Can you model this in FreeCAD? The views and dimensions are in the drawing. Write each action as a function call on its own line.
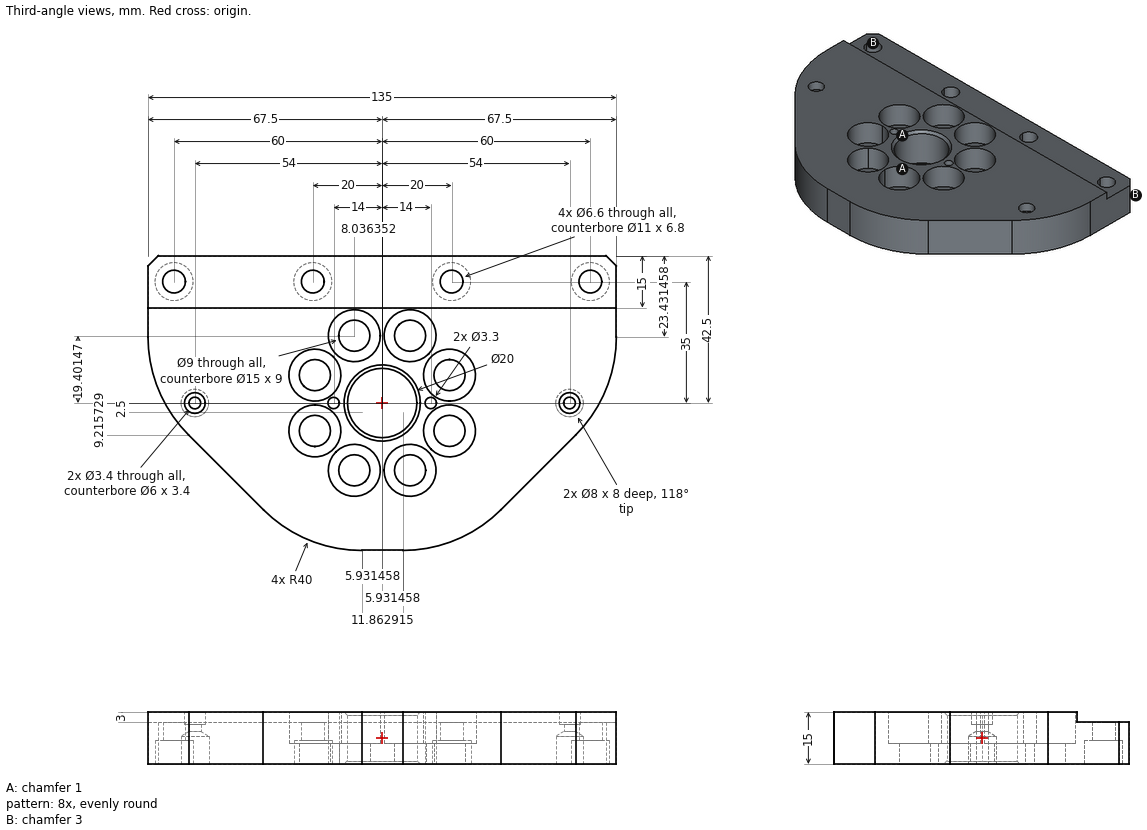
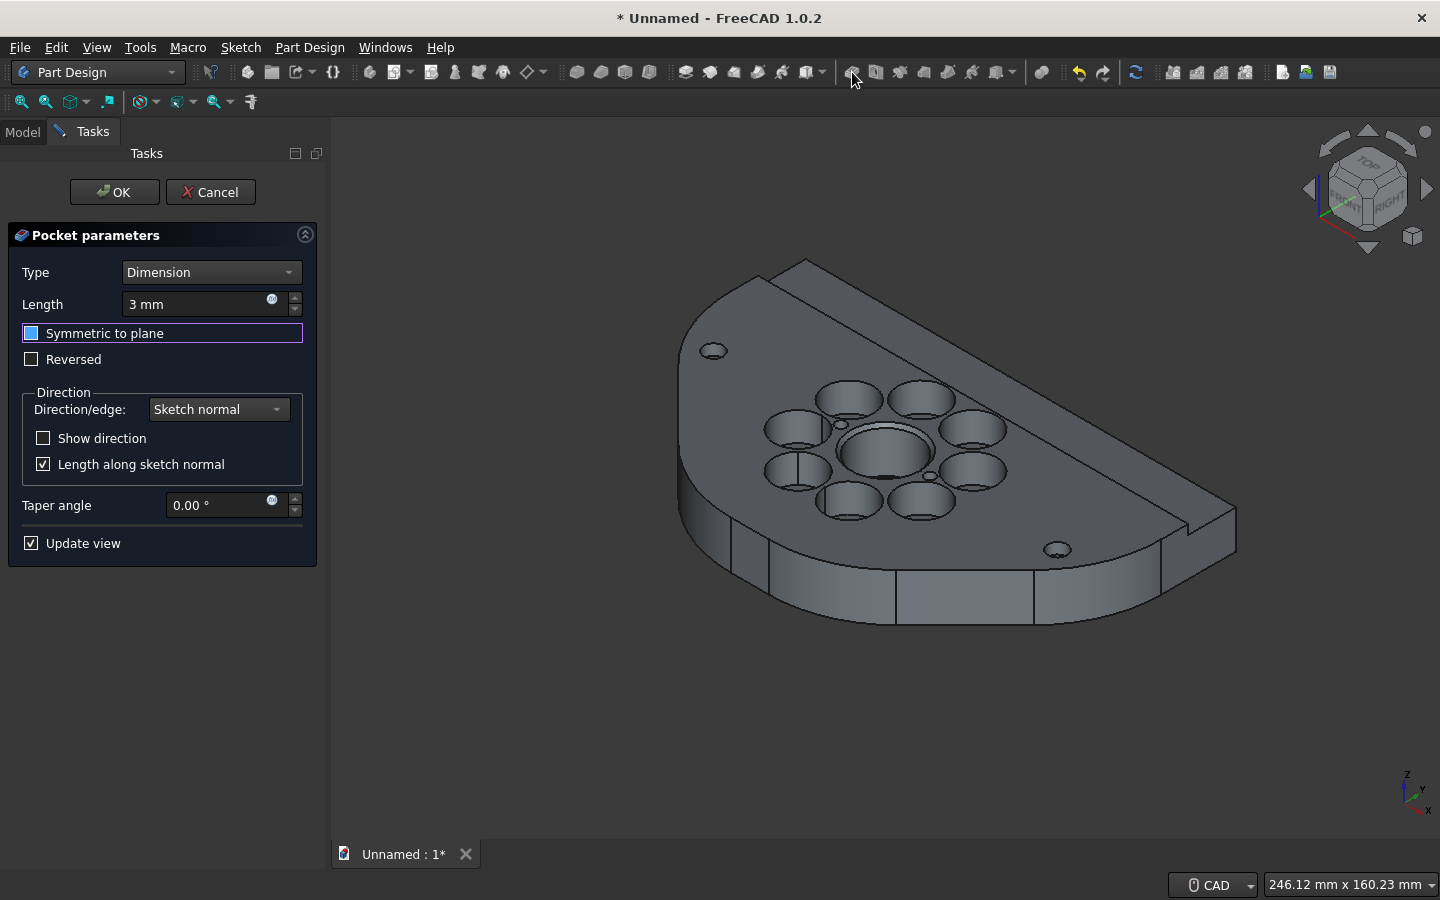
click(115, 192)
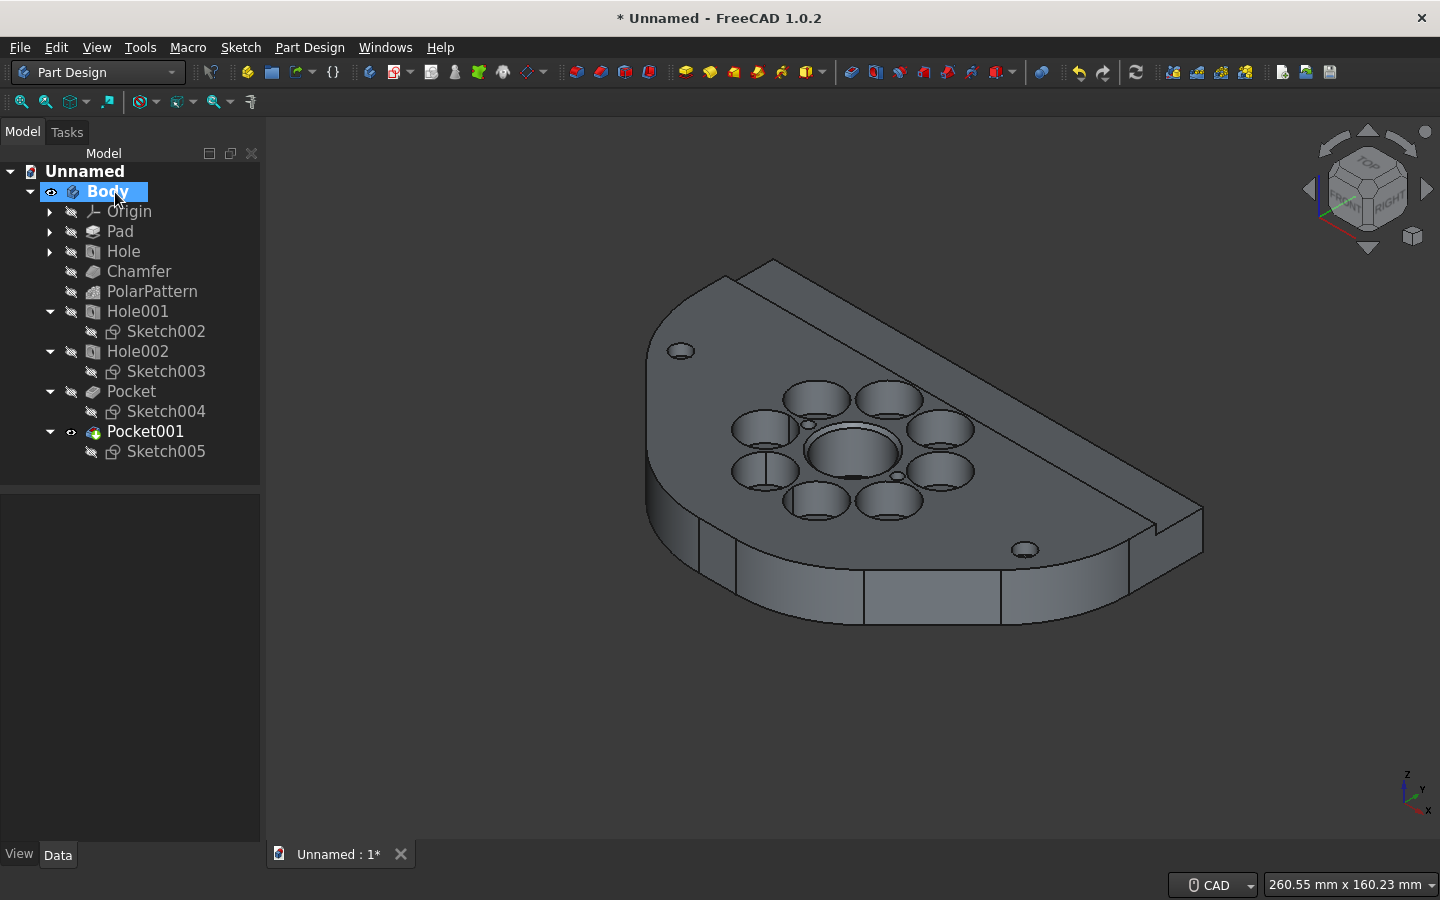
key(5)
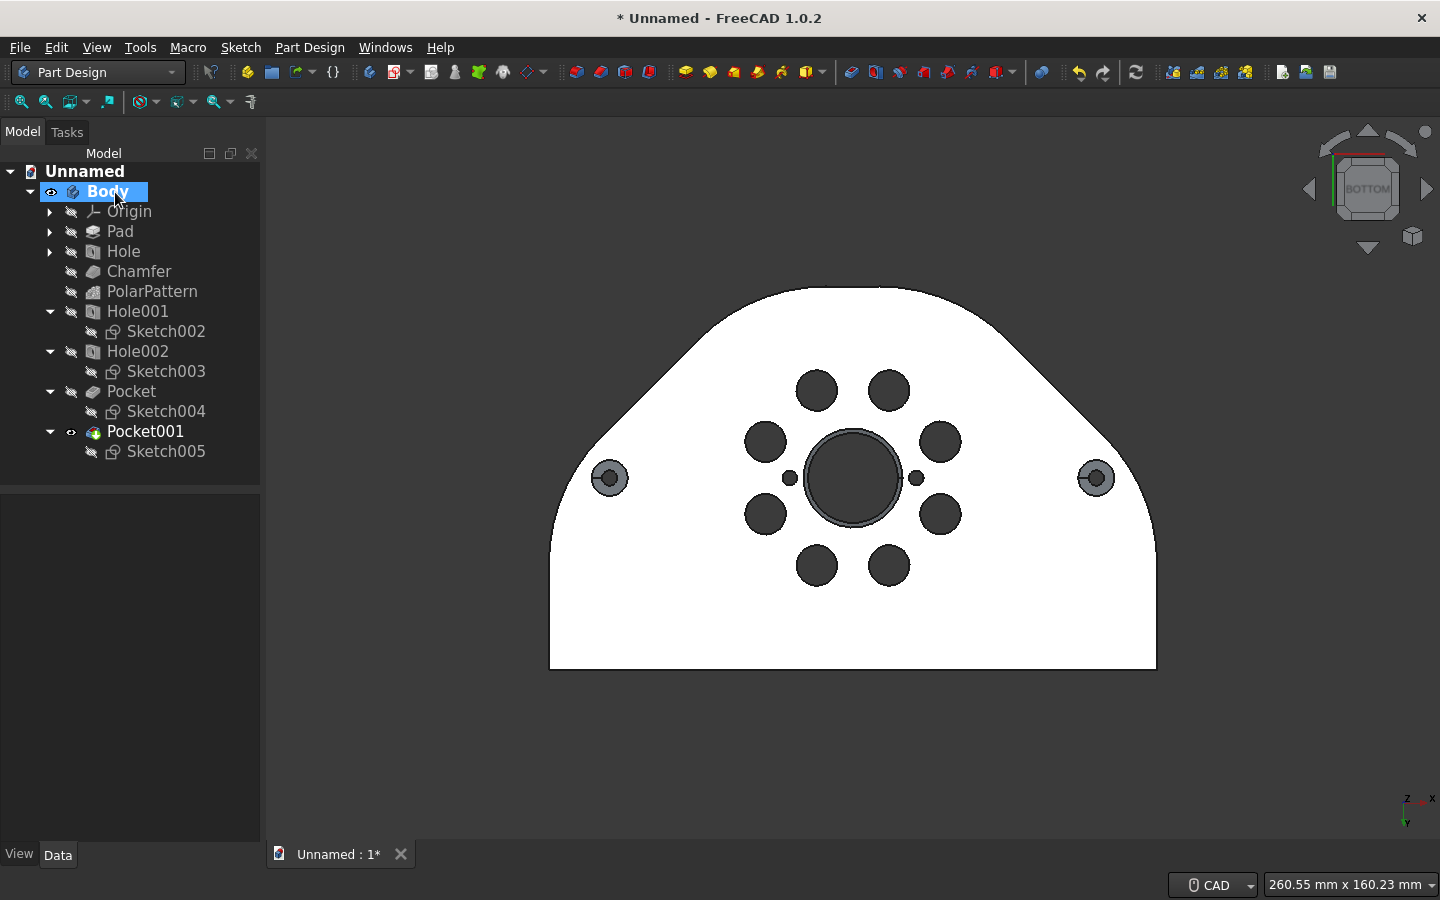
click(1027, 586)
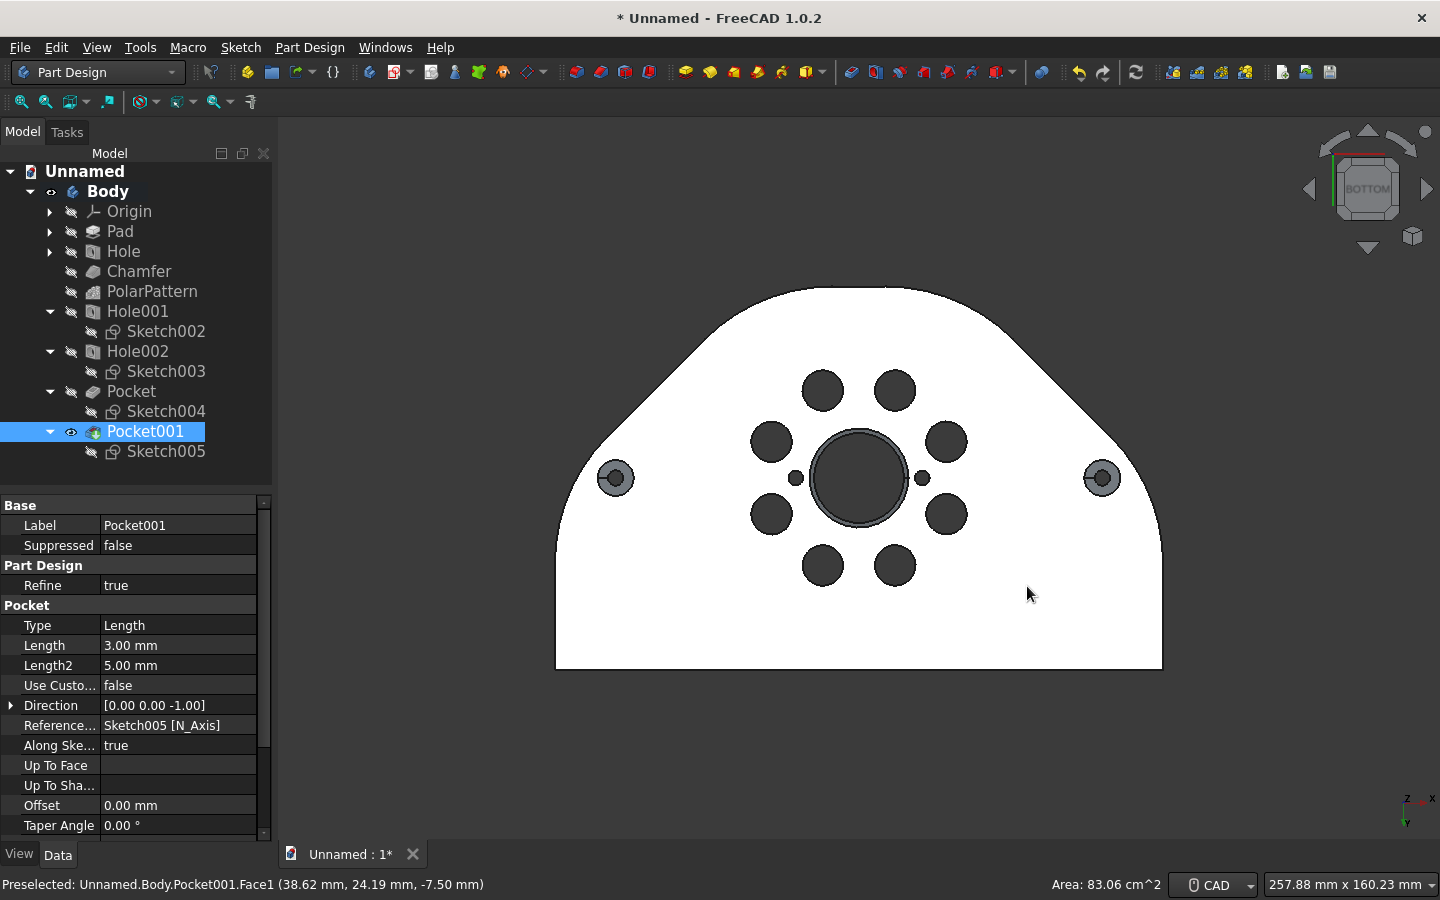
click(394, 72)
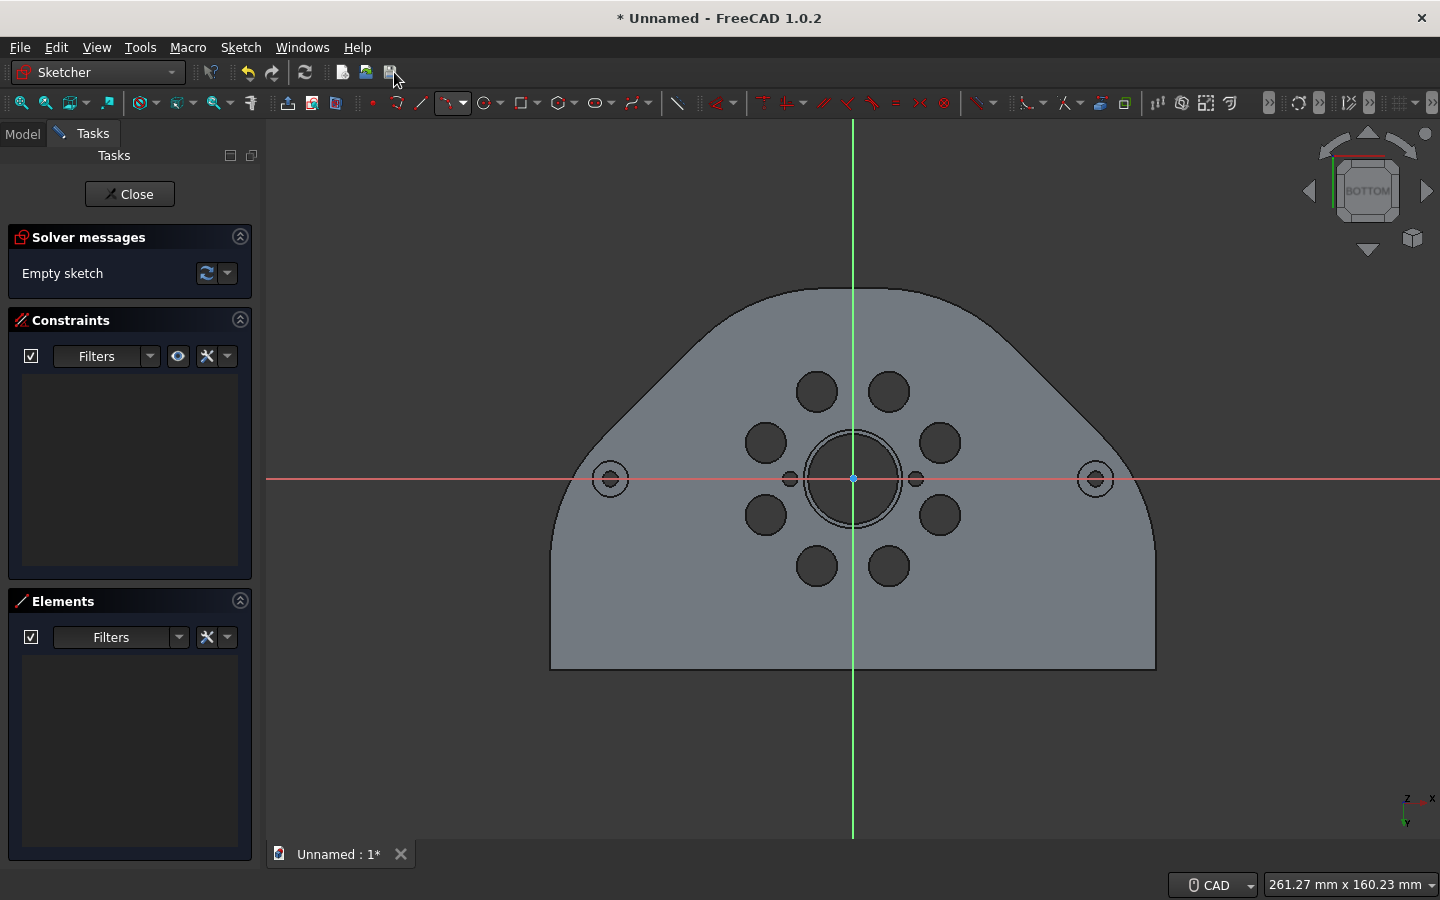
click(484, 104)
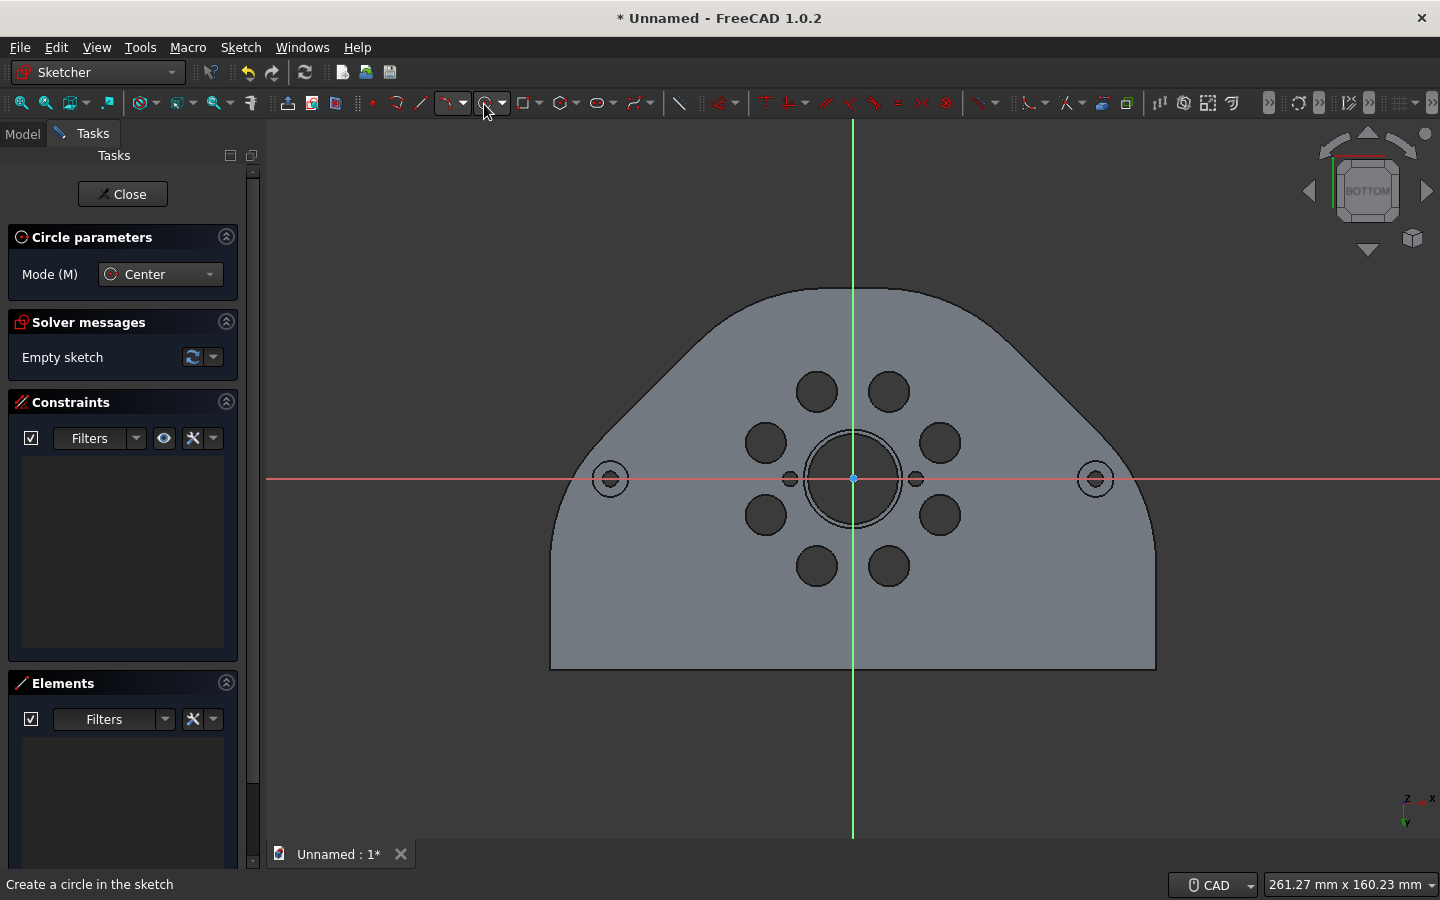
scroll(943, 636, up, 3)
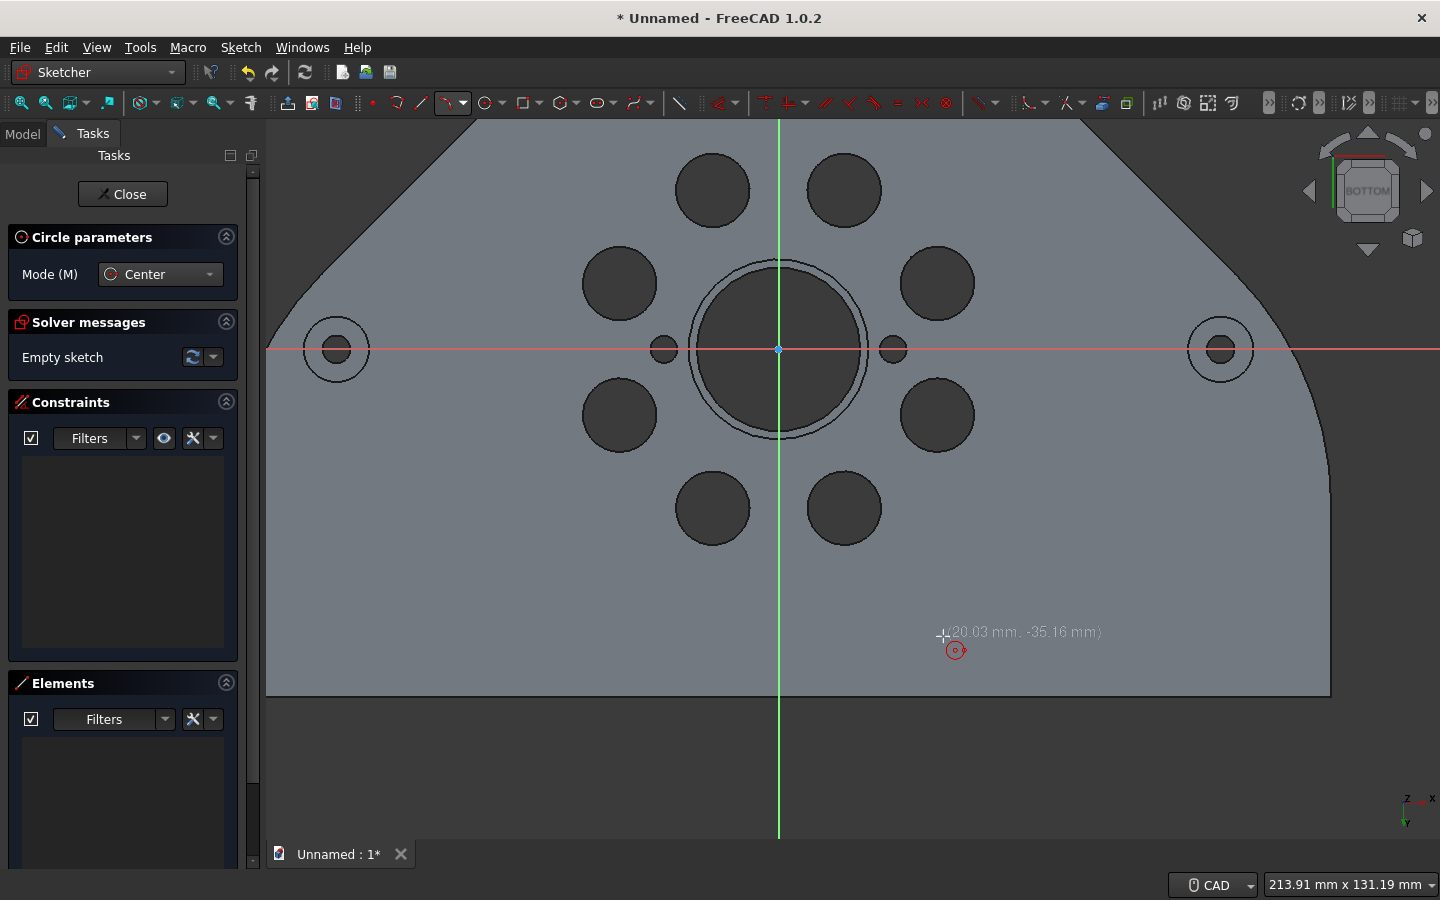
click(942, 636)
move(961, 617)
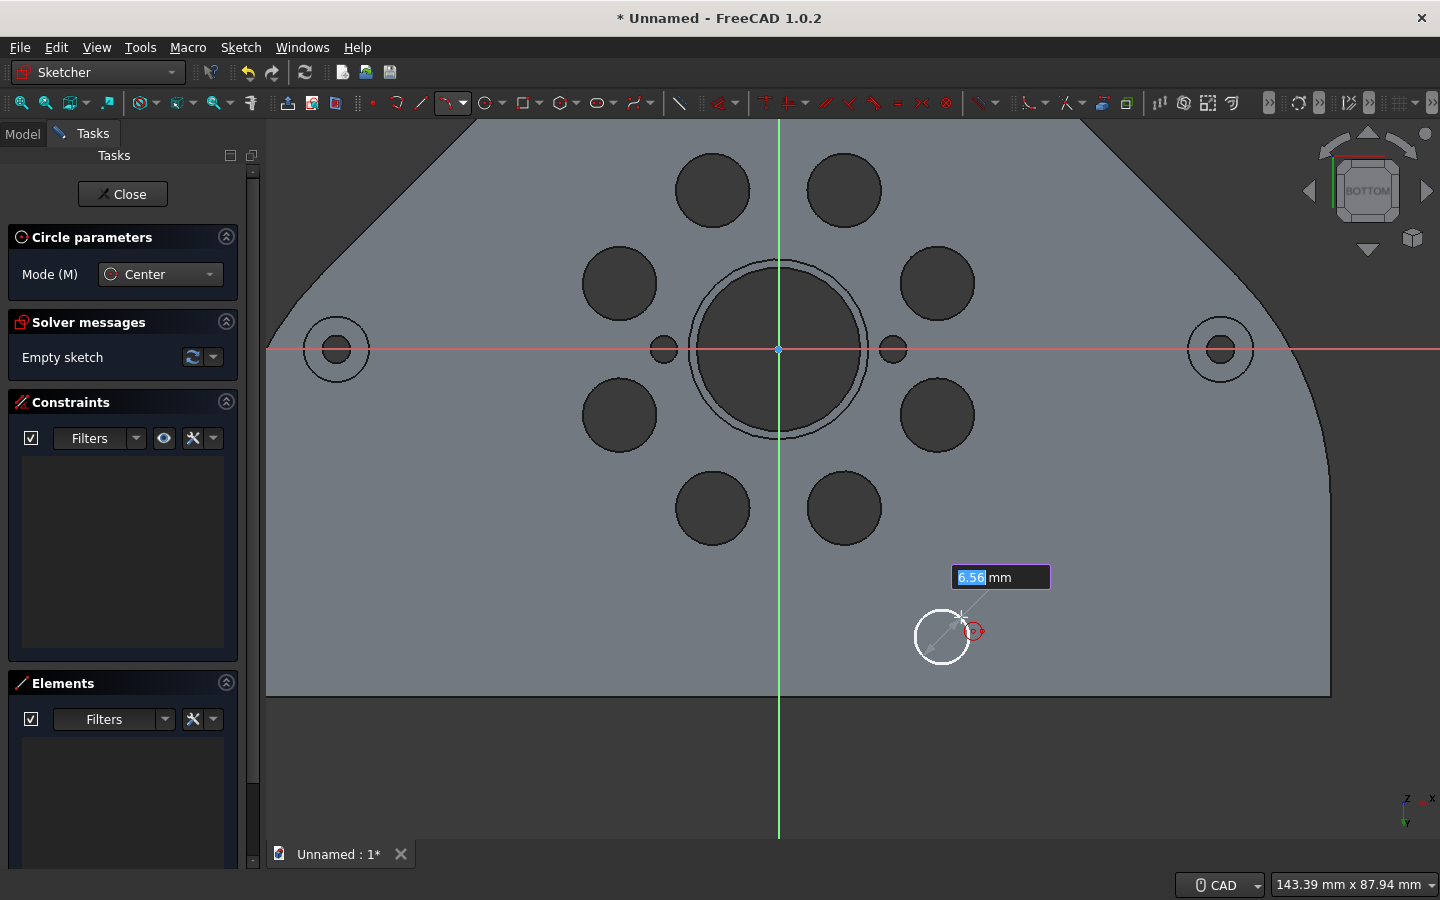
text(6.6)
key(Return)